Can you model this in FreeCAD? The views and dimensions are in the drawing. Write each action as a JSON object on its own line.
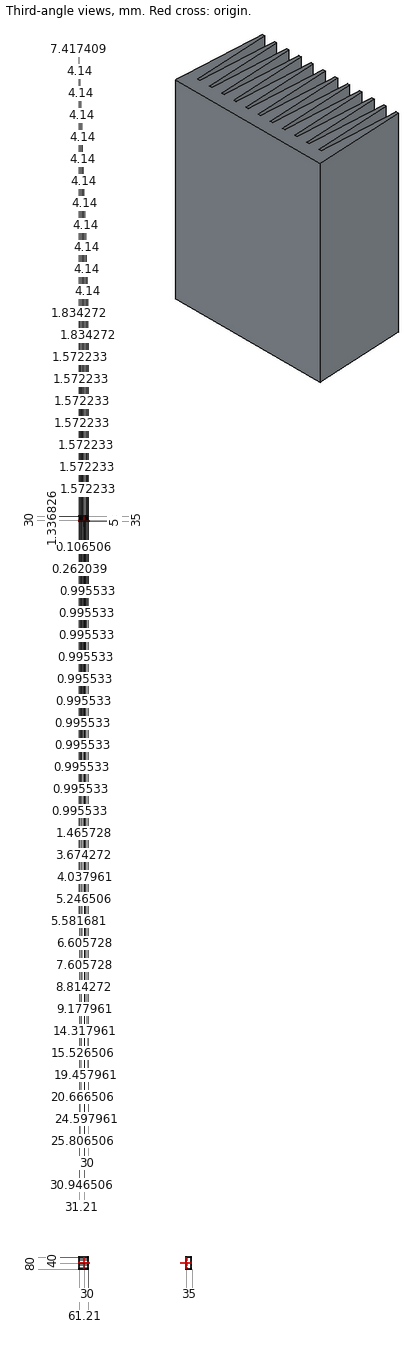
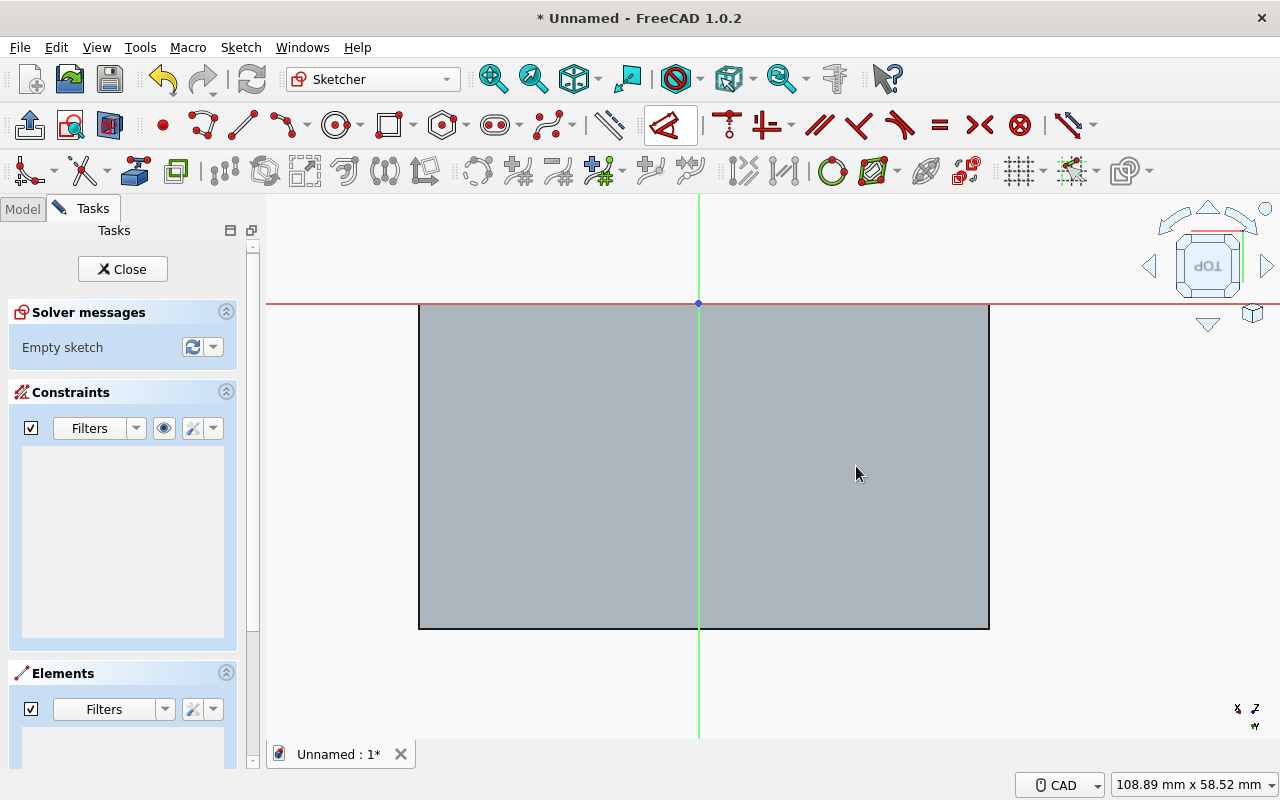
{"action": "left_click", "coordinate": [204, 126]}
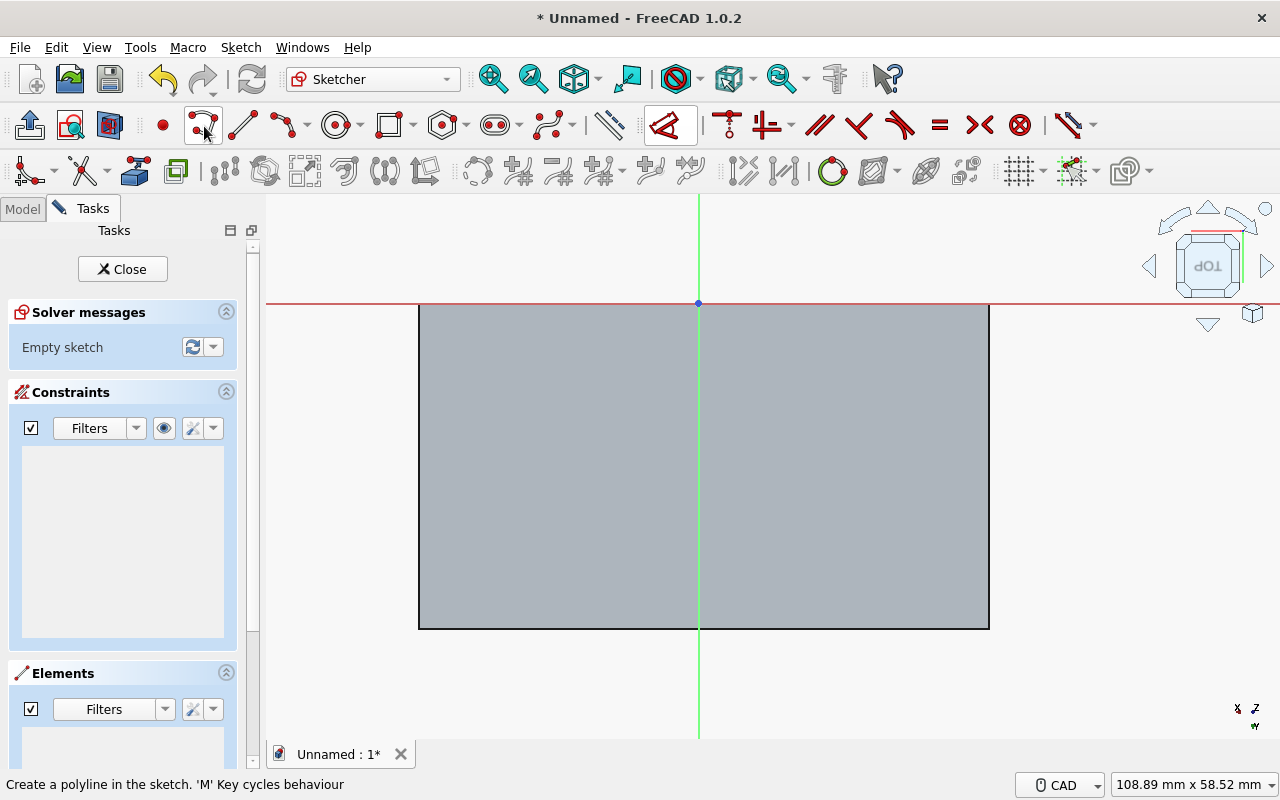
{"action": "left_click", "coordinate": [470, 350]}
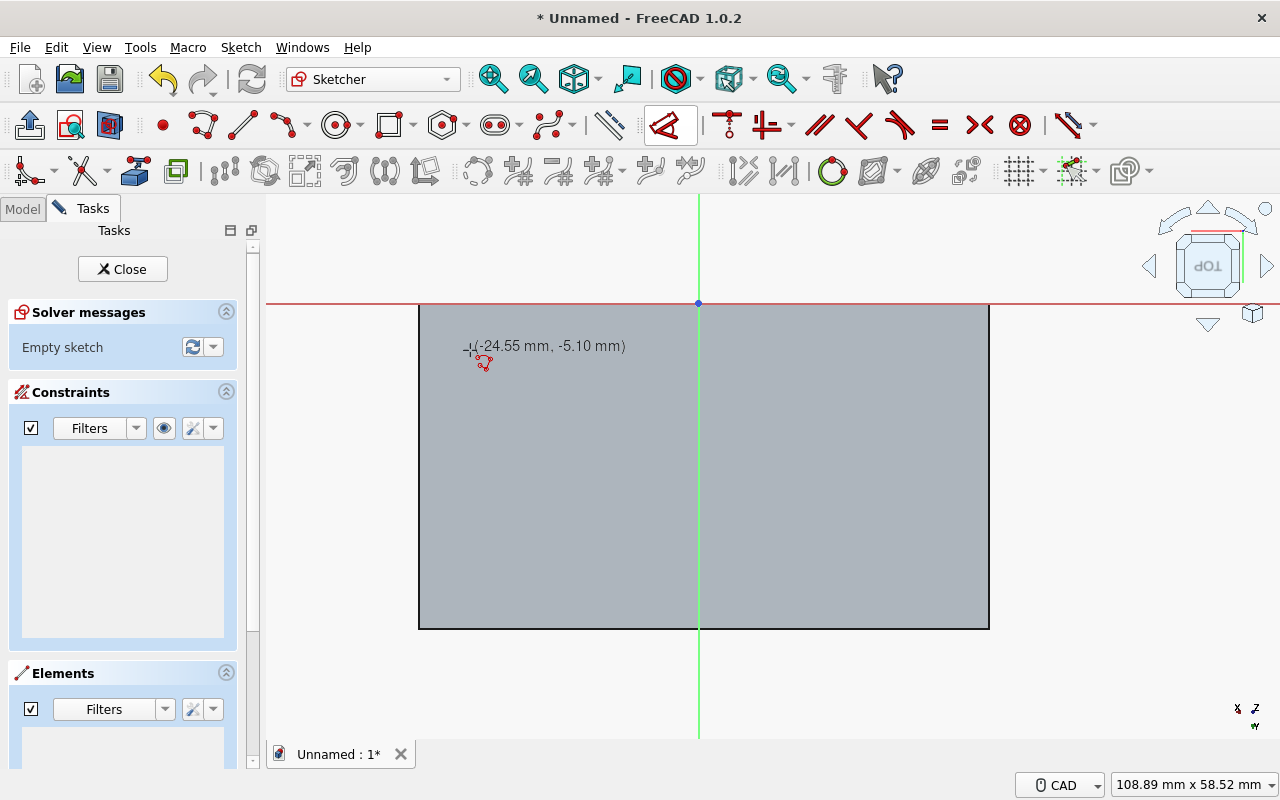
{"action": "scroll", "coordinate": [460, 350], "scroll_direction": "up", "scroll_amount": 3}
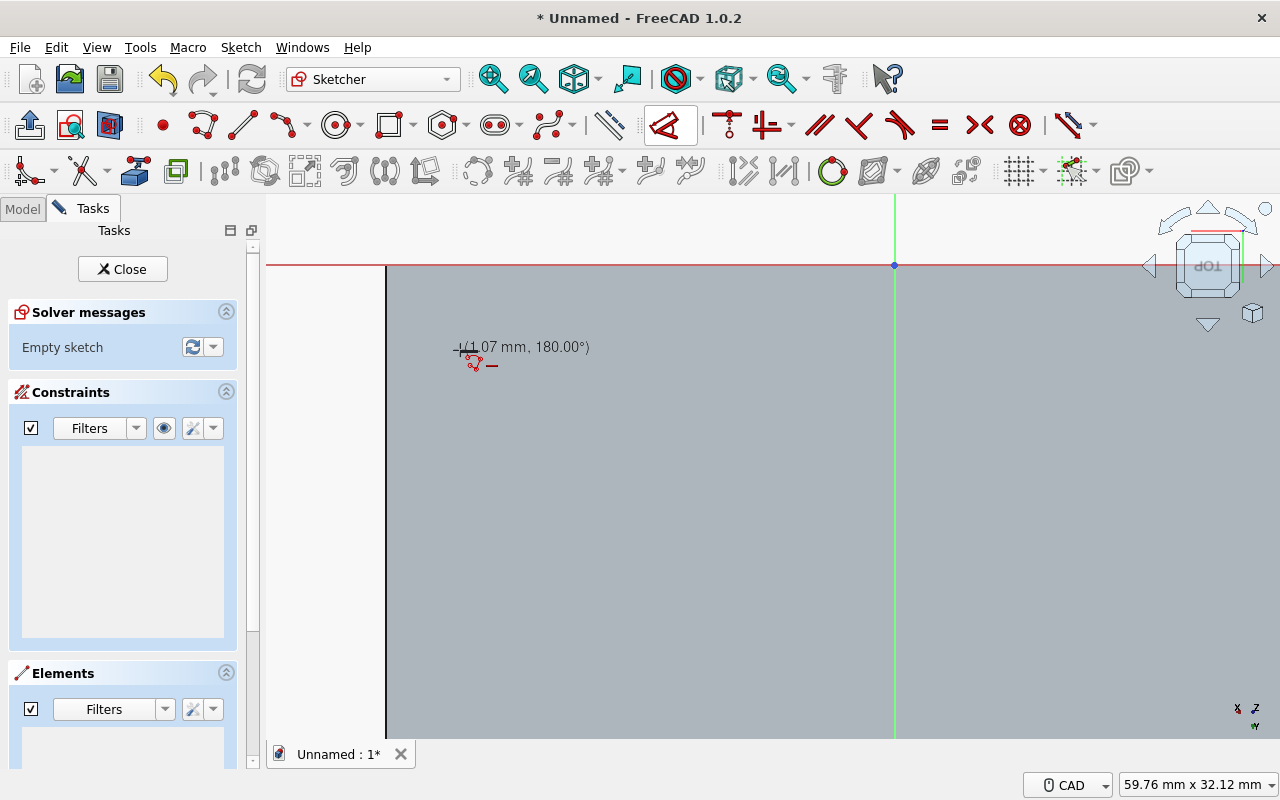
{"action": "left_click", "coordinate": [460, 350]}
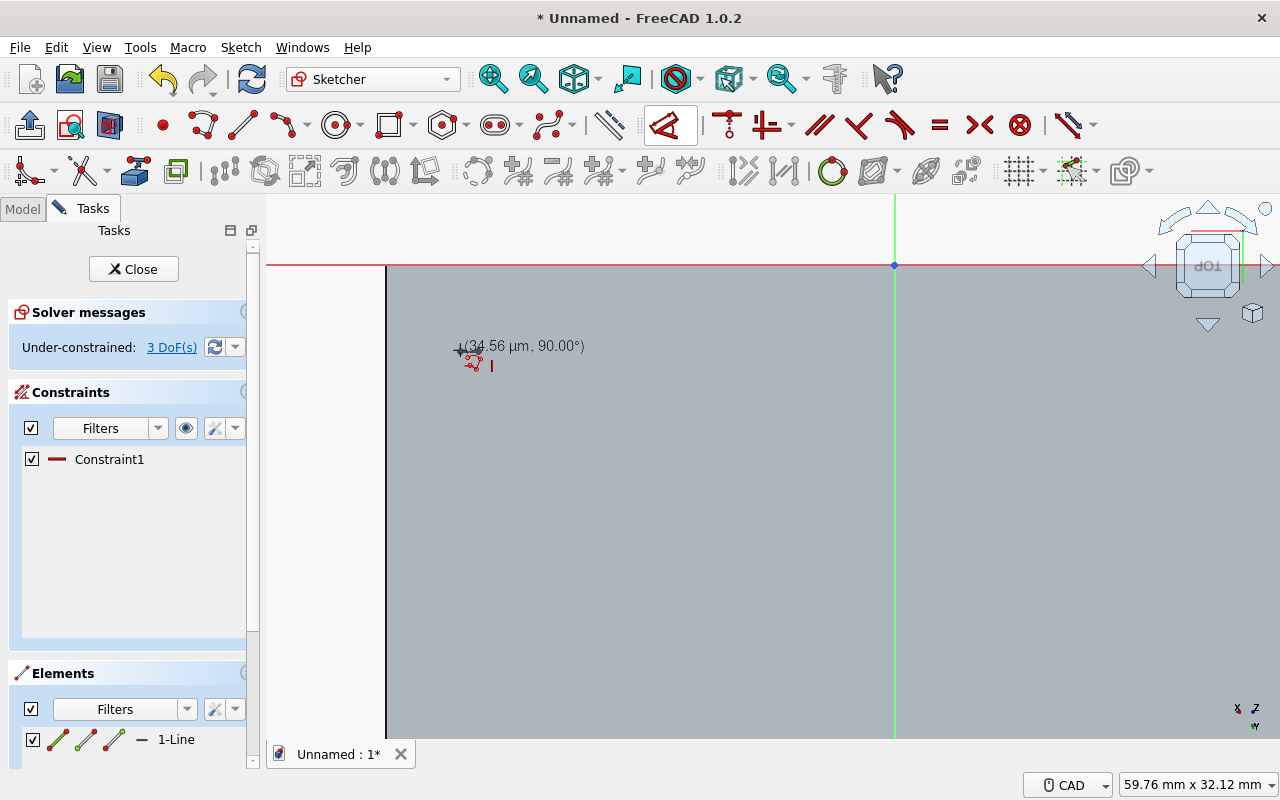
{"action": "scroll", "coordinate": [461, 350], "scroll_direction": "down", "scroll_amount": 3}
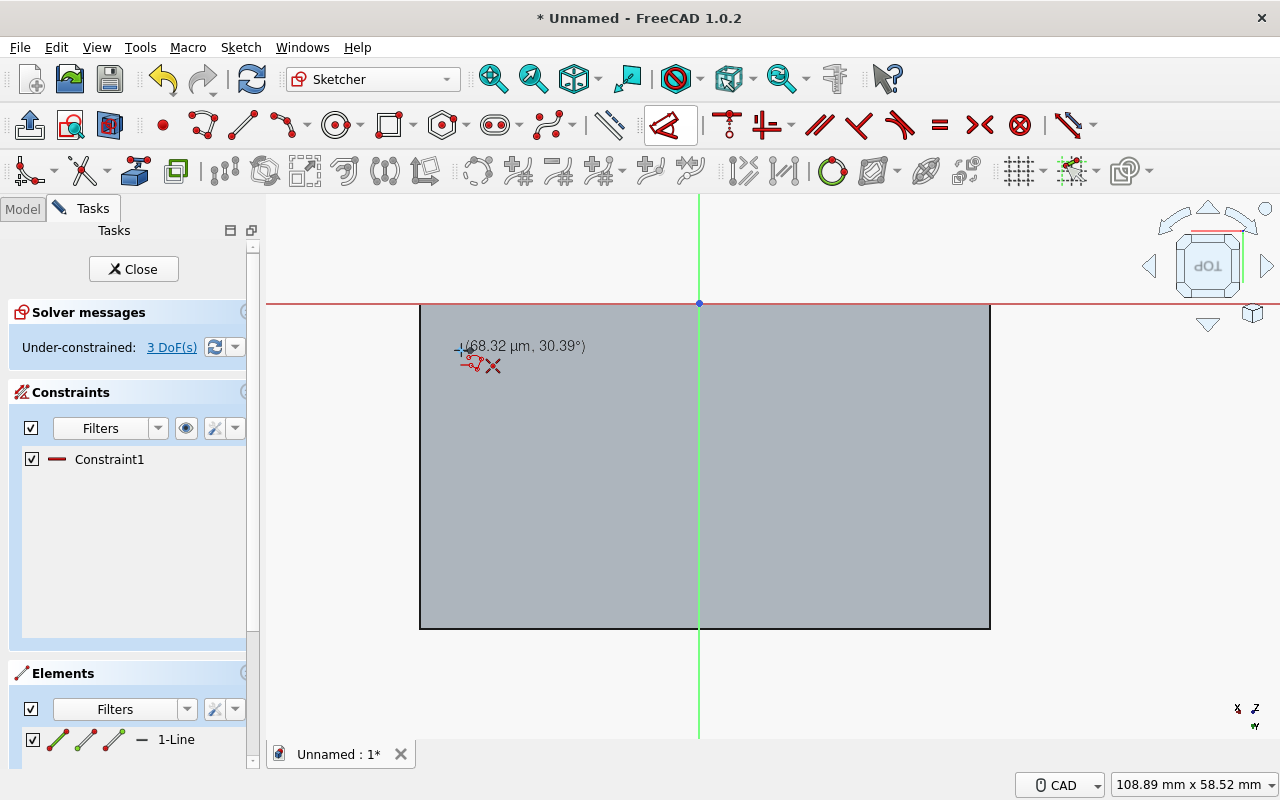
{"action": "left_click", "coordinate": [446, 629]}
{"action": "left_click", "coordinate": [485, 629]}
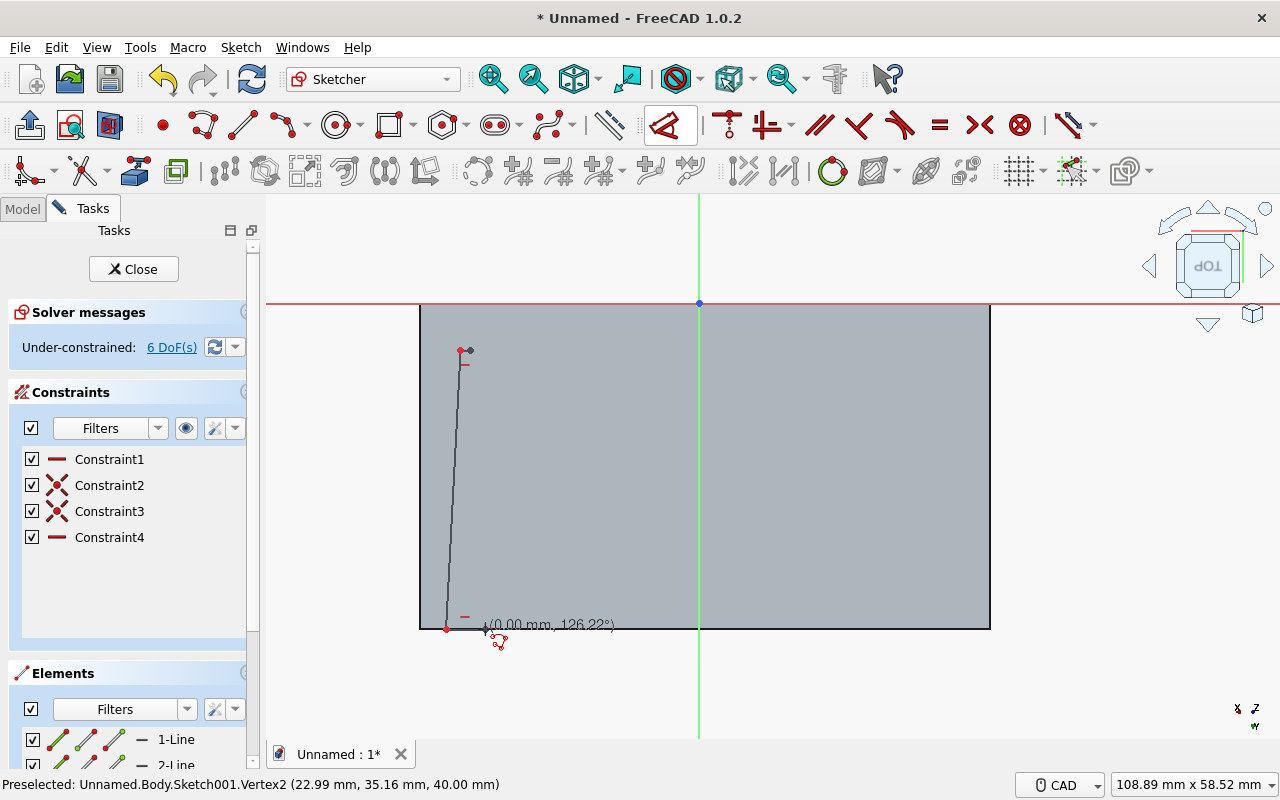
{"action": "scroll", "coordinate": [470, 350], "scroll_direction": "up", "scroll_amount": 7}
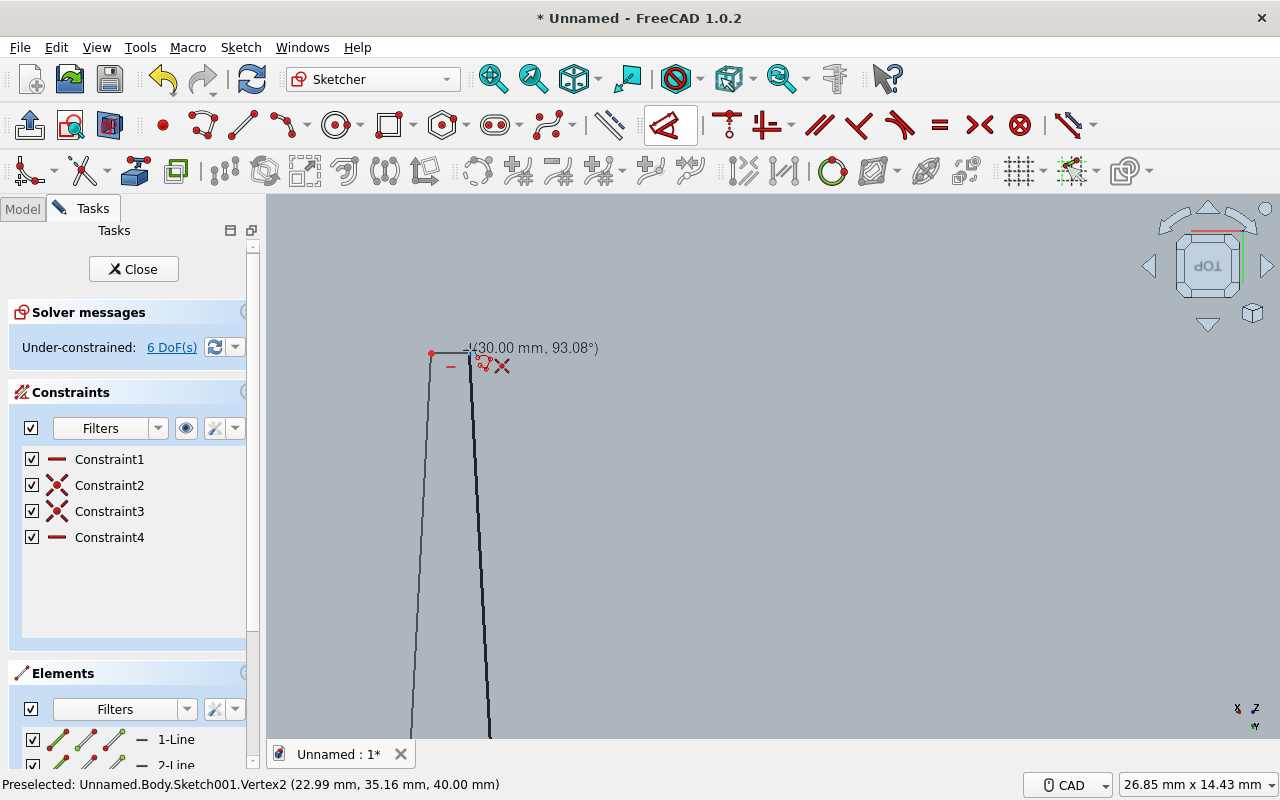
{"action": "left_click", "coordinate": [471, 353]}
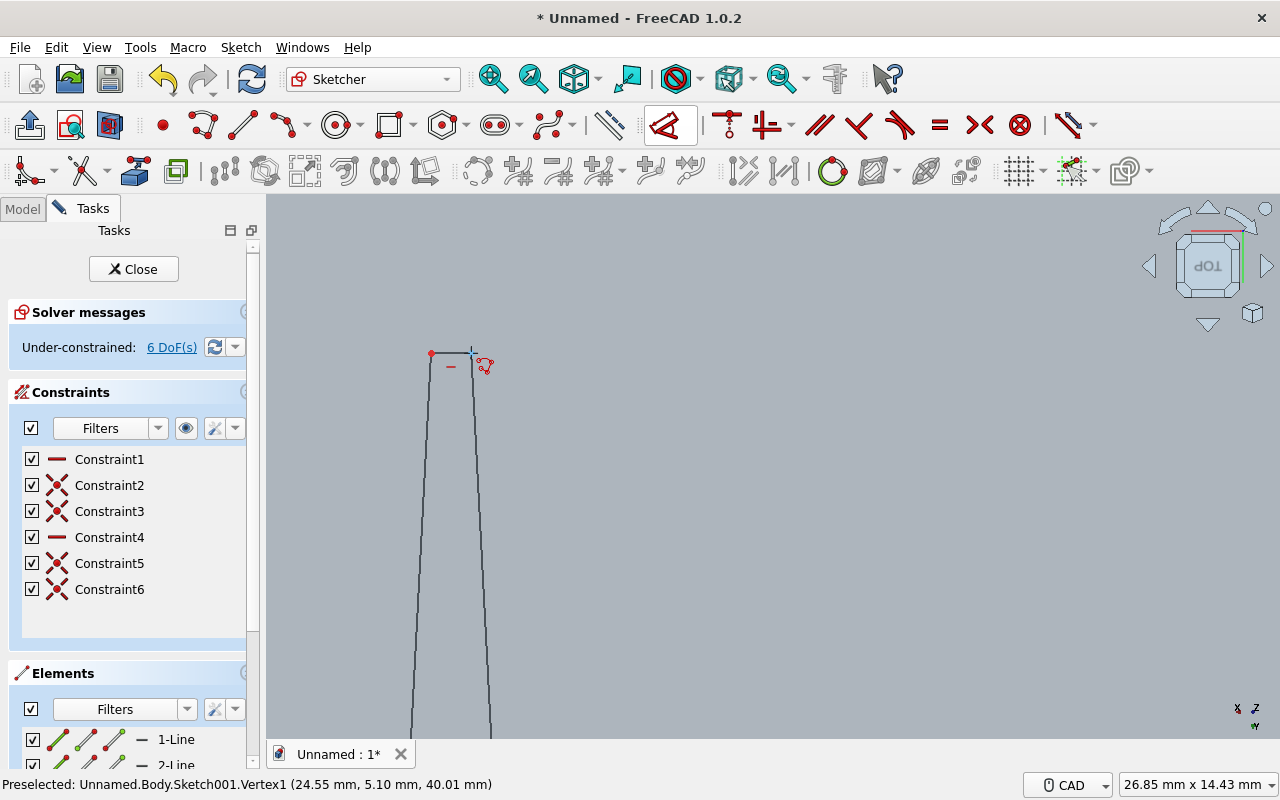
{"action": "scroll", "coordinate": [470, 350], "scroll_direction": "down", "scroll_amount": 7}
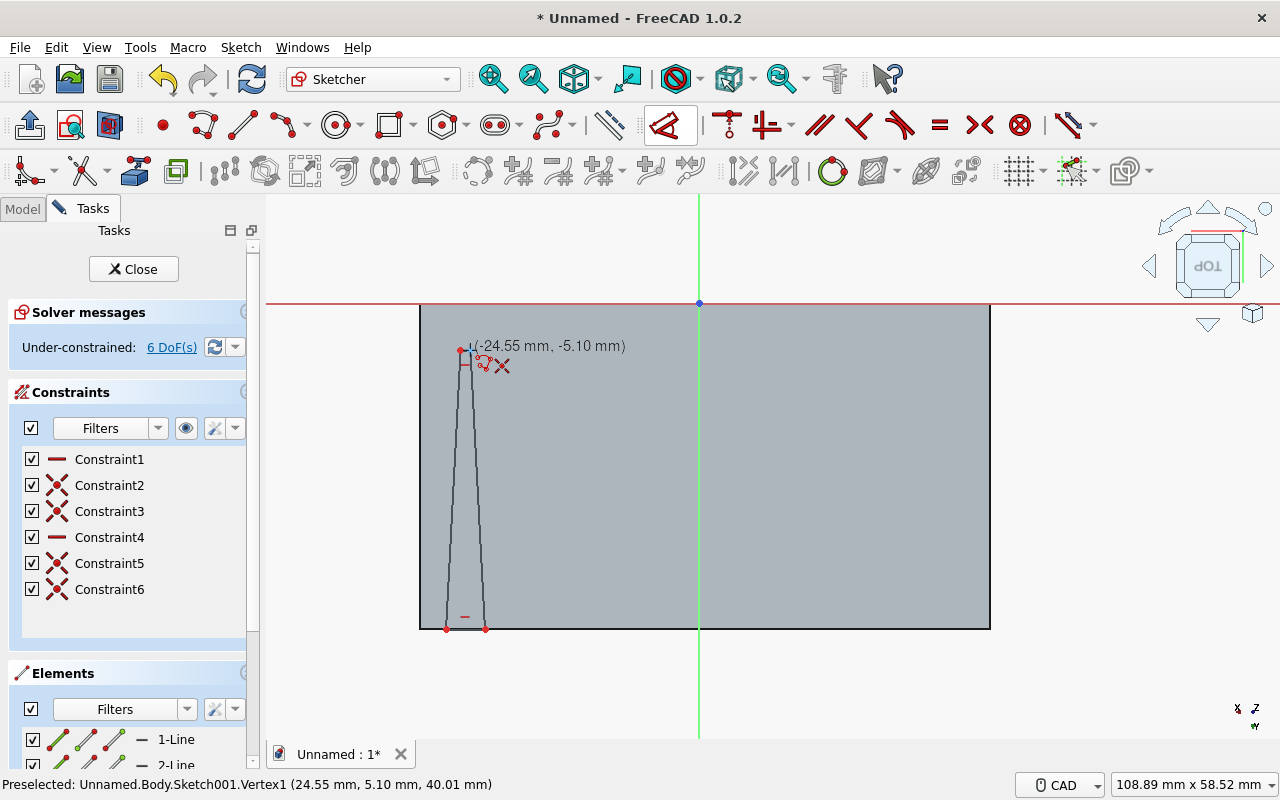
{"action": "left_click", "coordinate": [420, 304]}
{"action": "left_click", "coordinate": [420, 629]}